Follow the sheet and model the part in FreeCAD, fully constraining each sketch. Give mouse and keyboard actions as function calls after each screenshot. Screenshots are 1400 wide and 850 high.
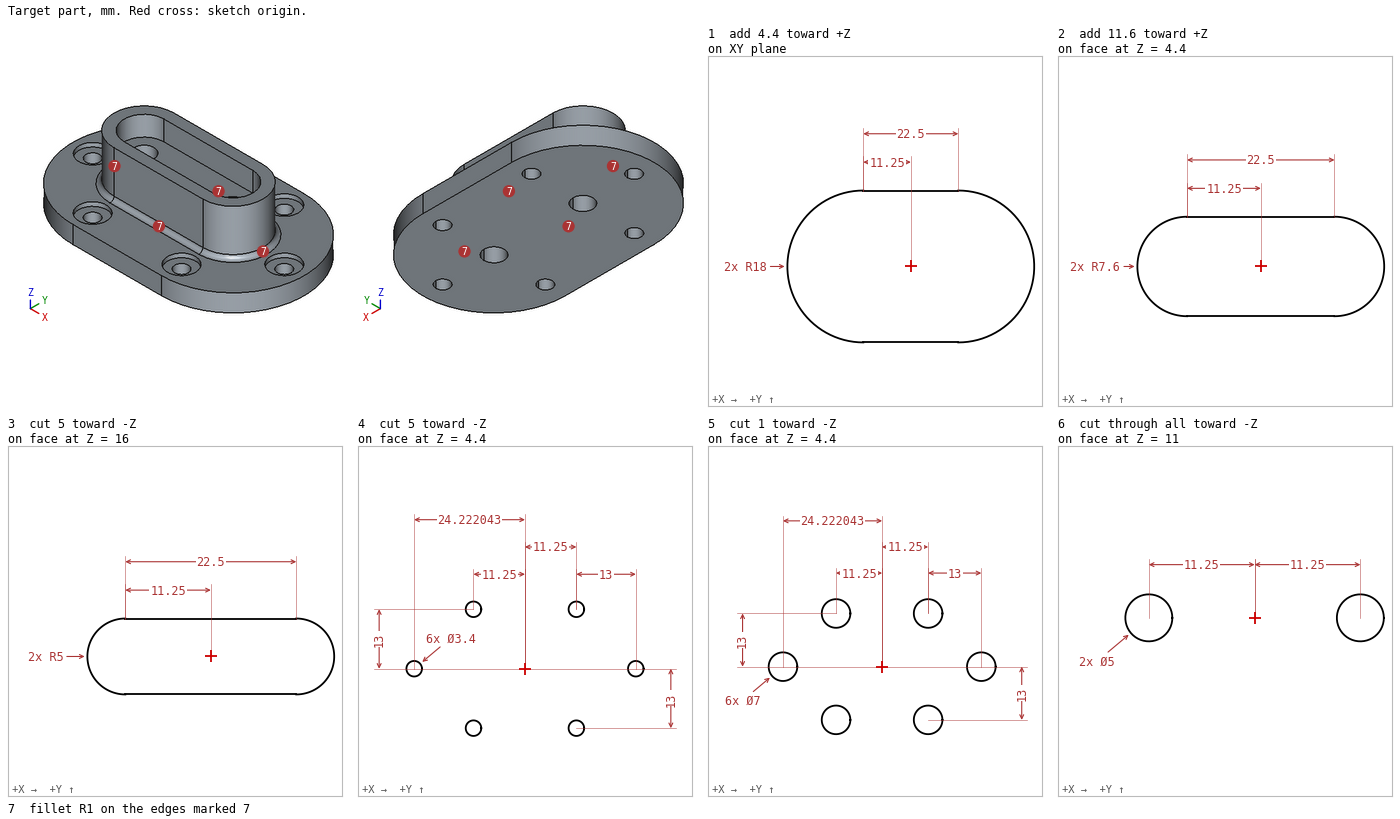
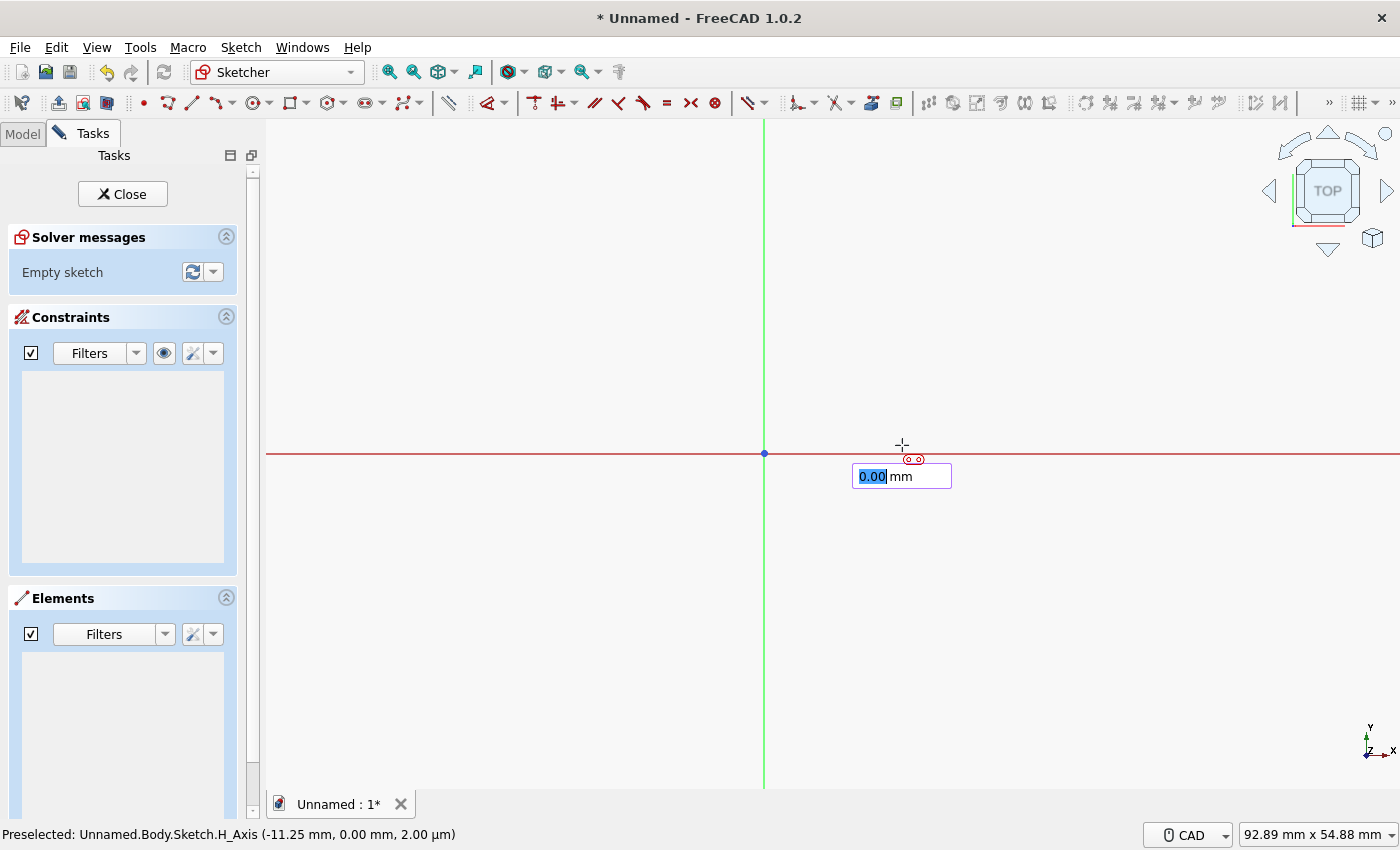
click(805, 234)
key(Escape)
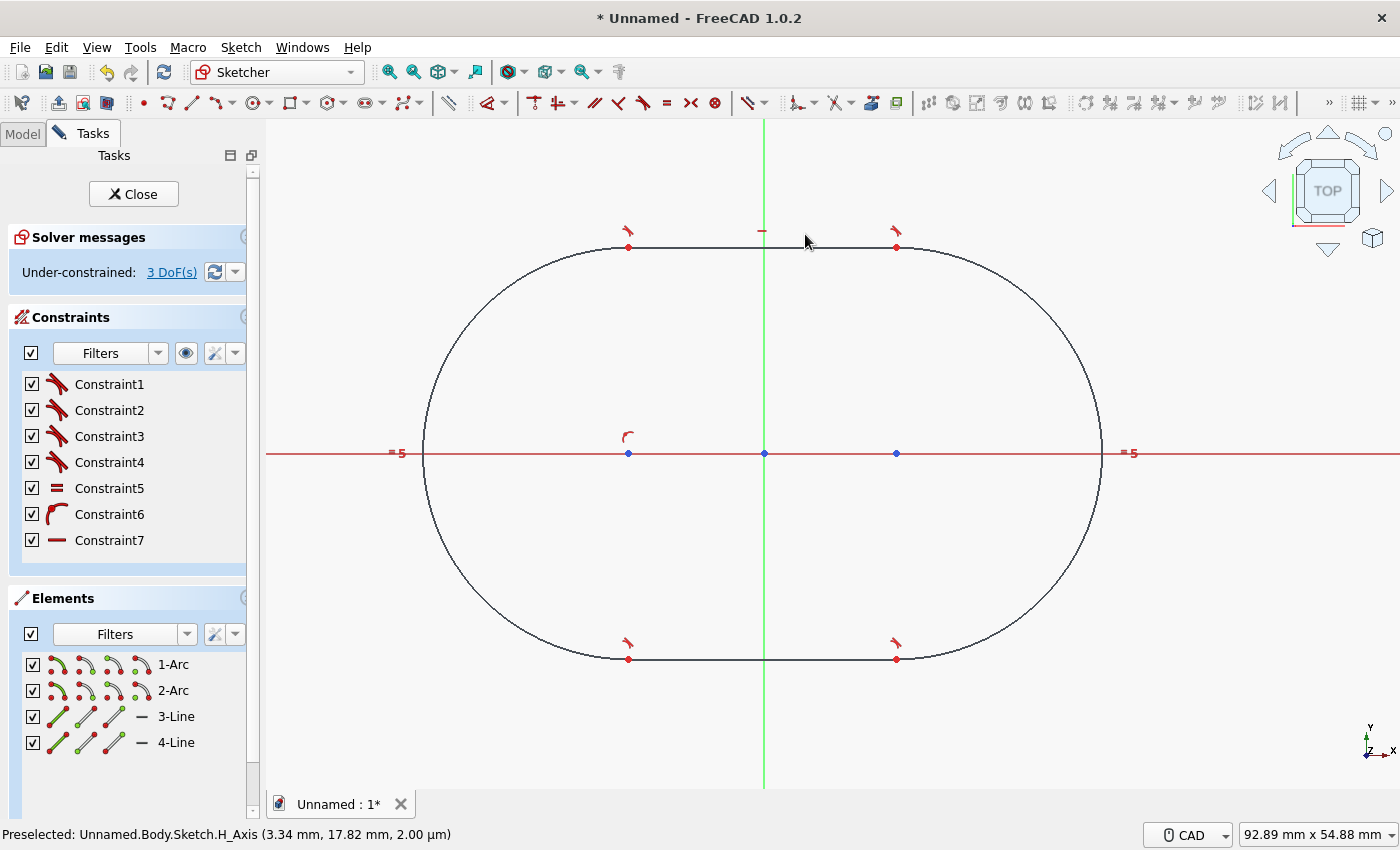
click(488, 104)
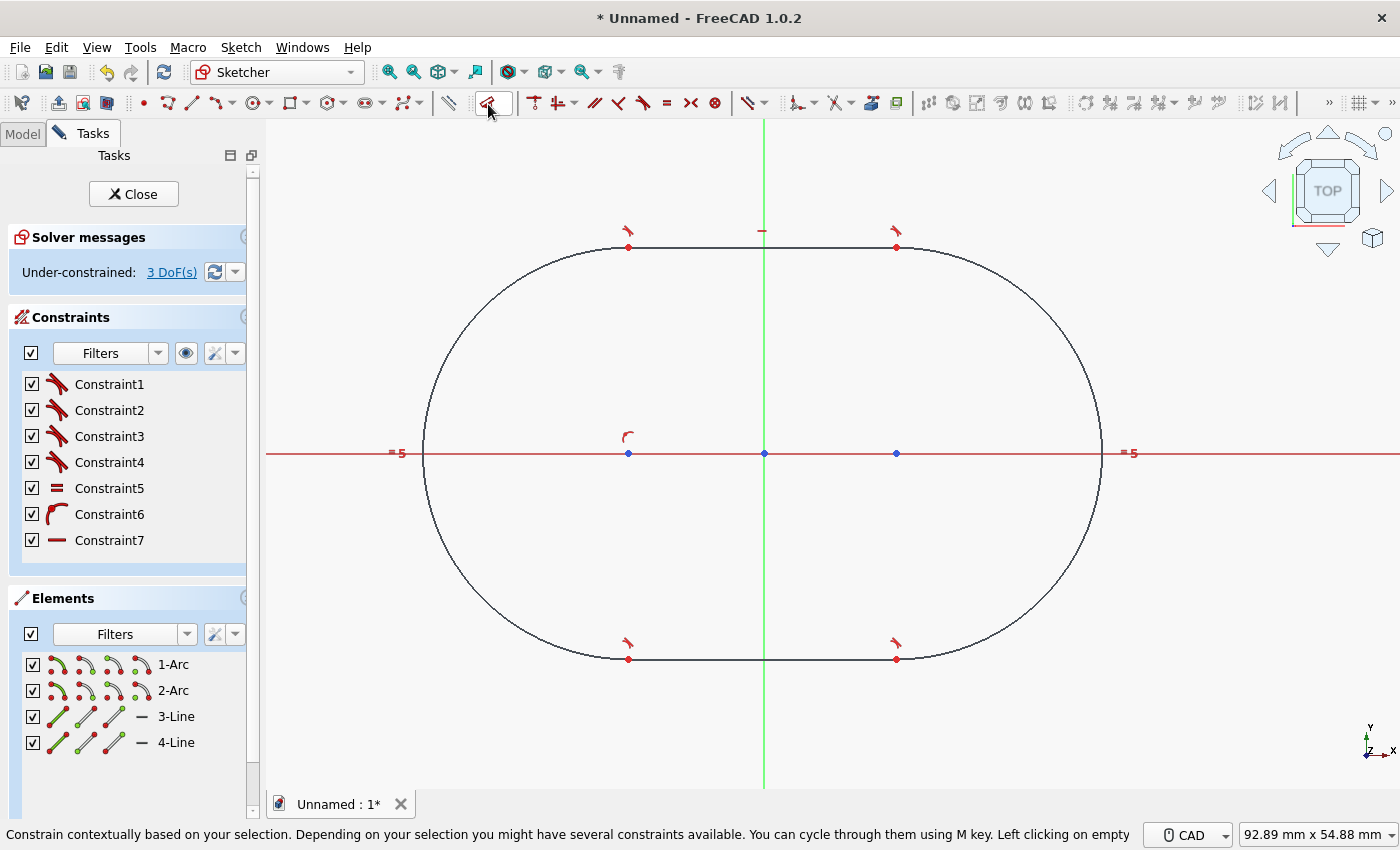
click(462, 333)
click(436, 314)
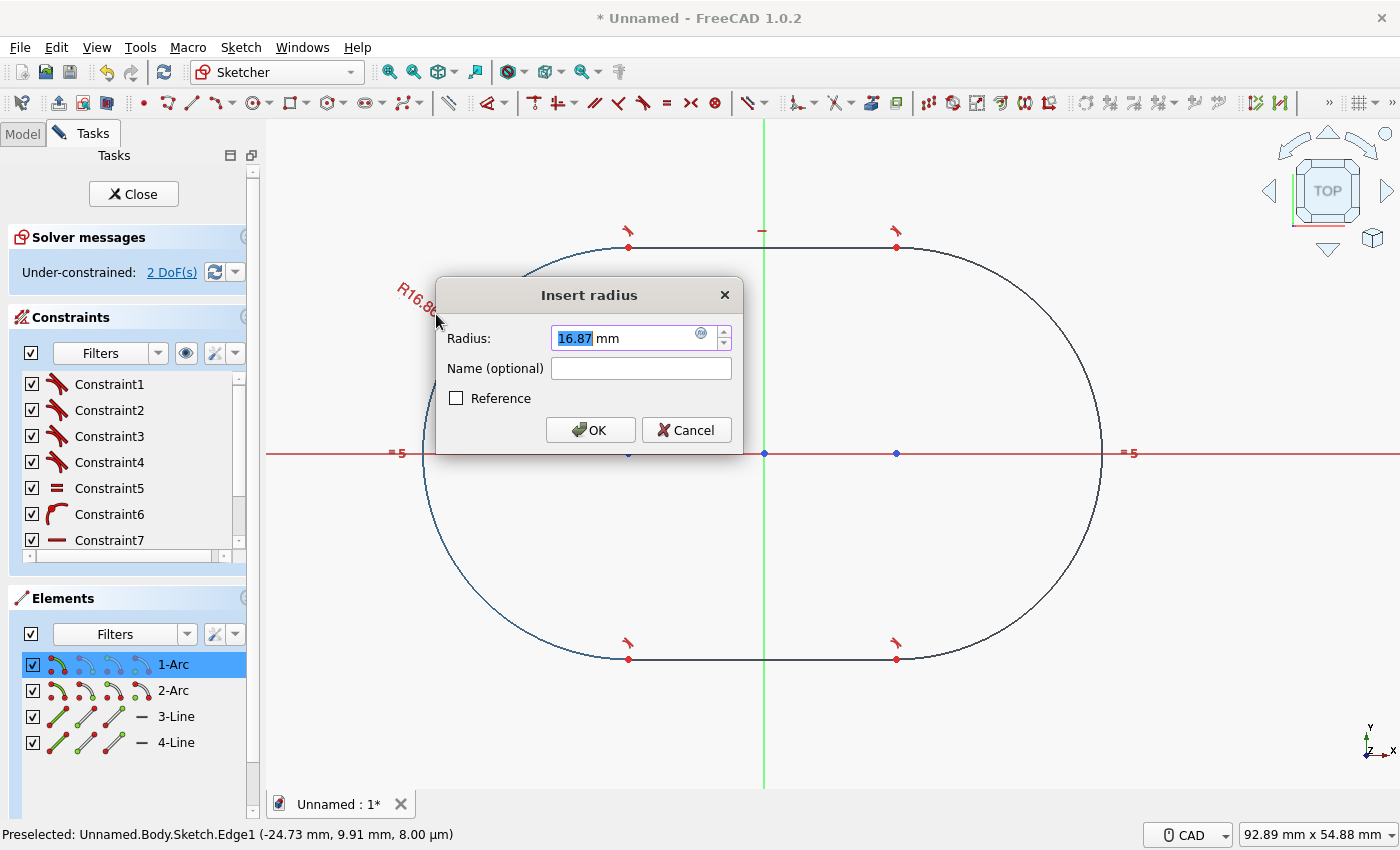
text(18)
key(Return)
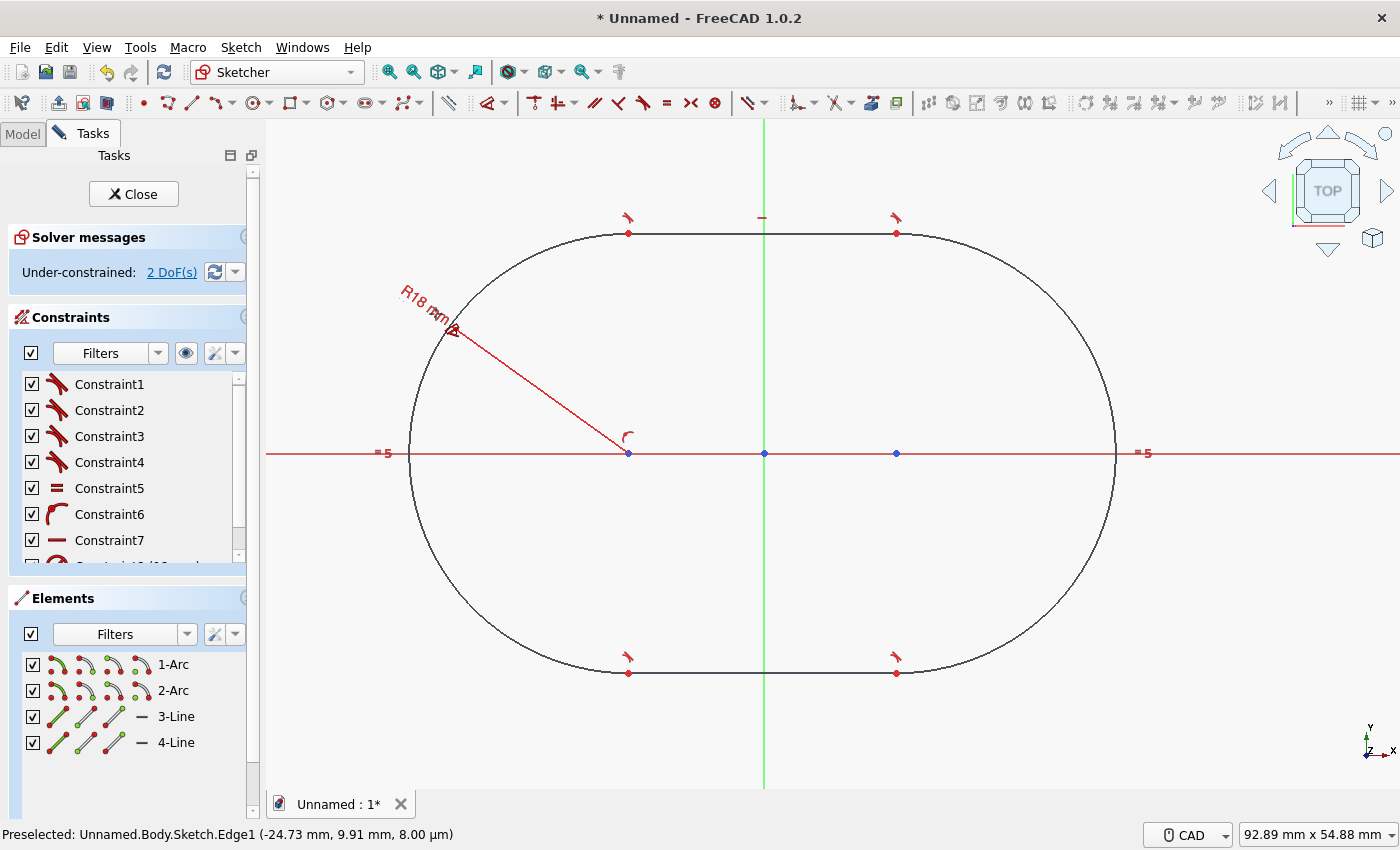
click(709, 234)
click(701, 200)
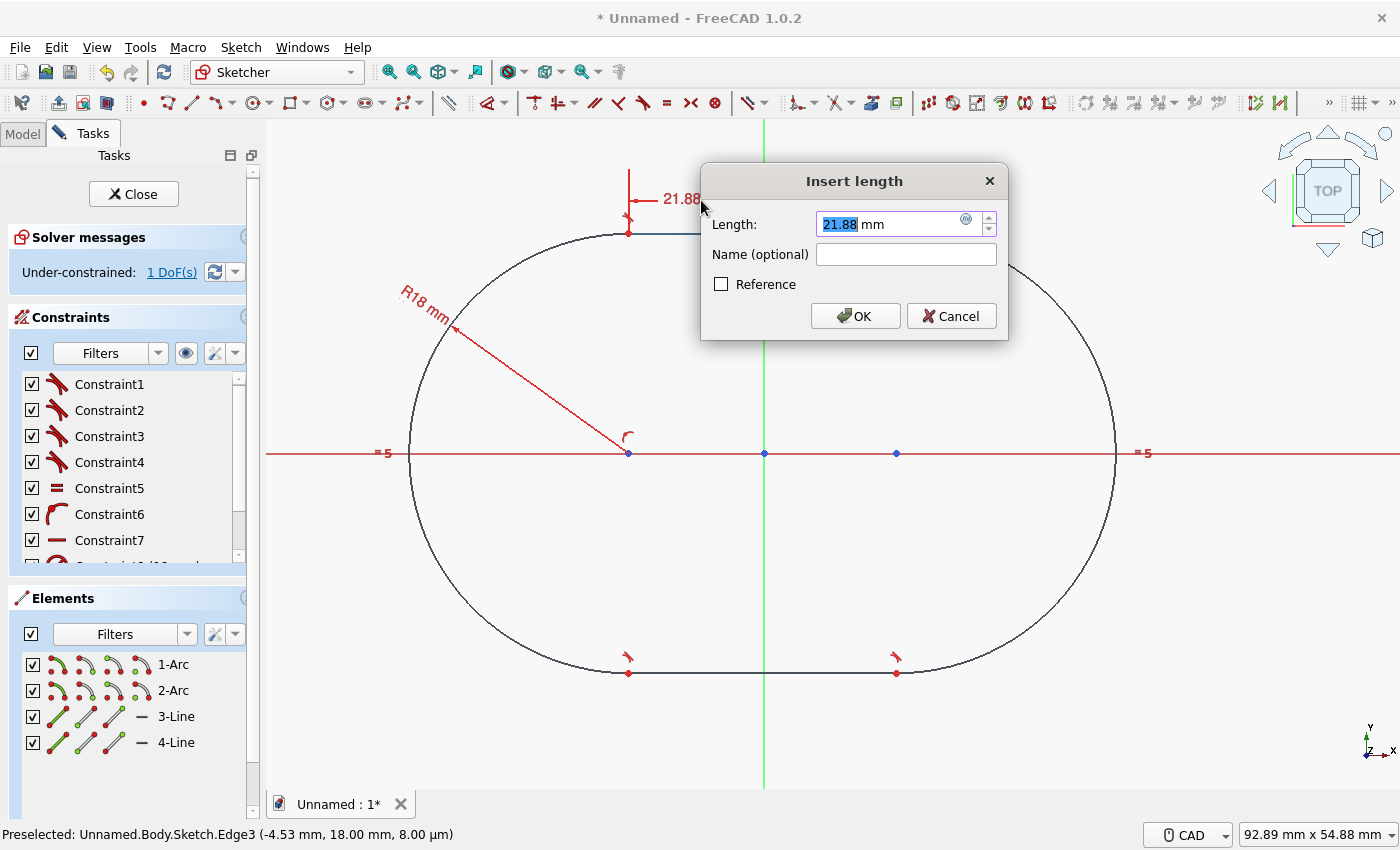
text(22.5)
key(Return)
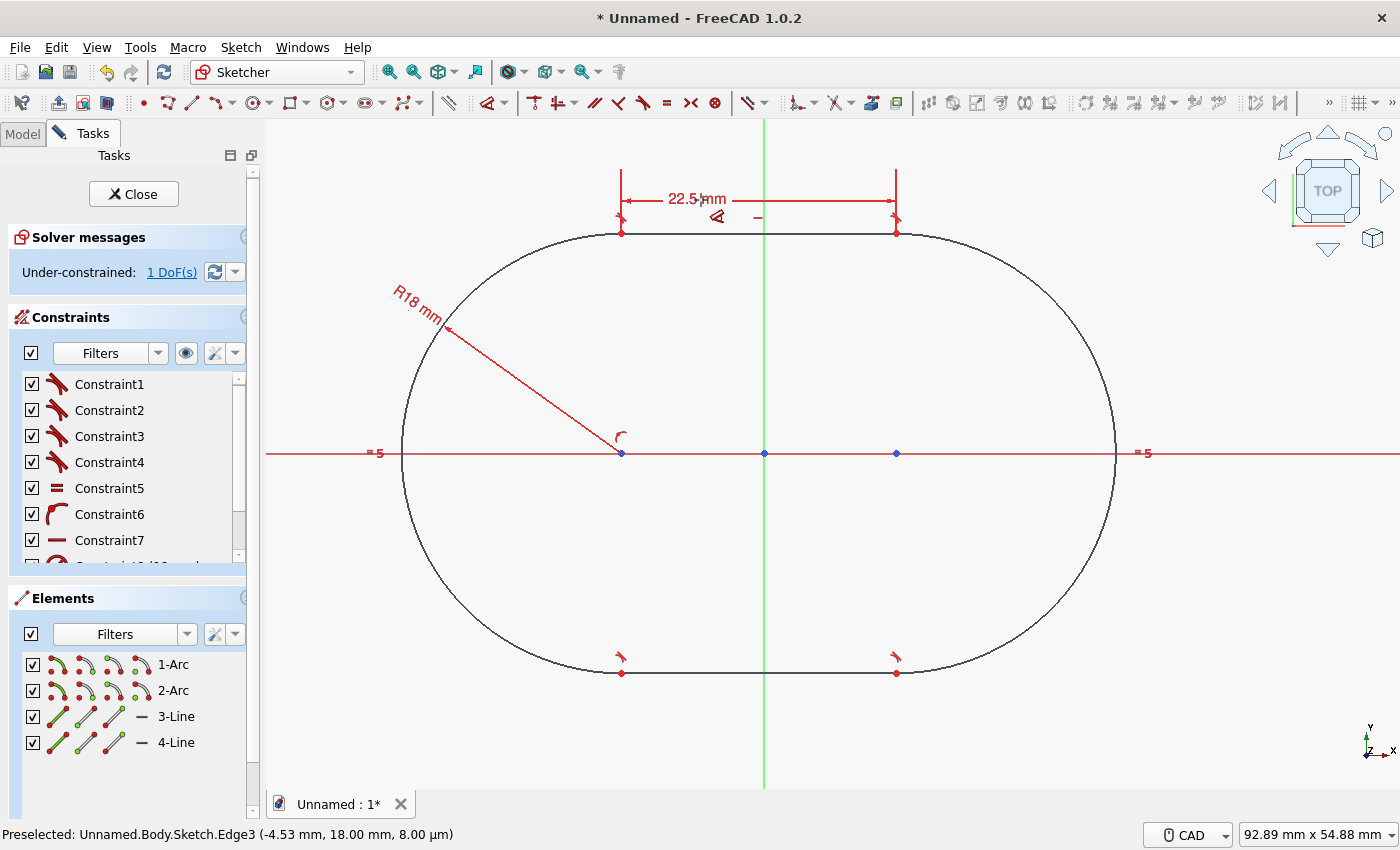
click(621, 234)
click(693, 488)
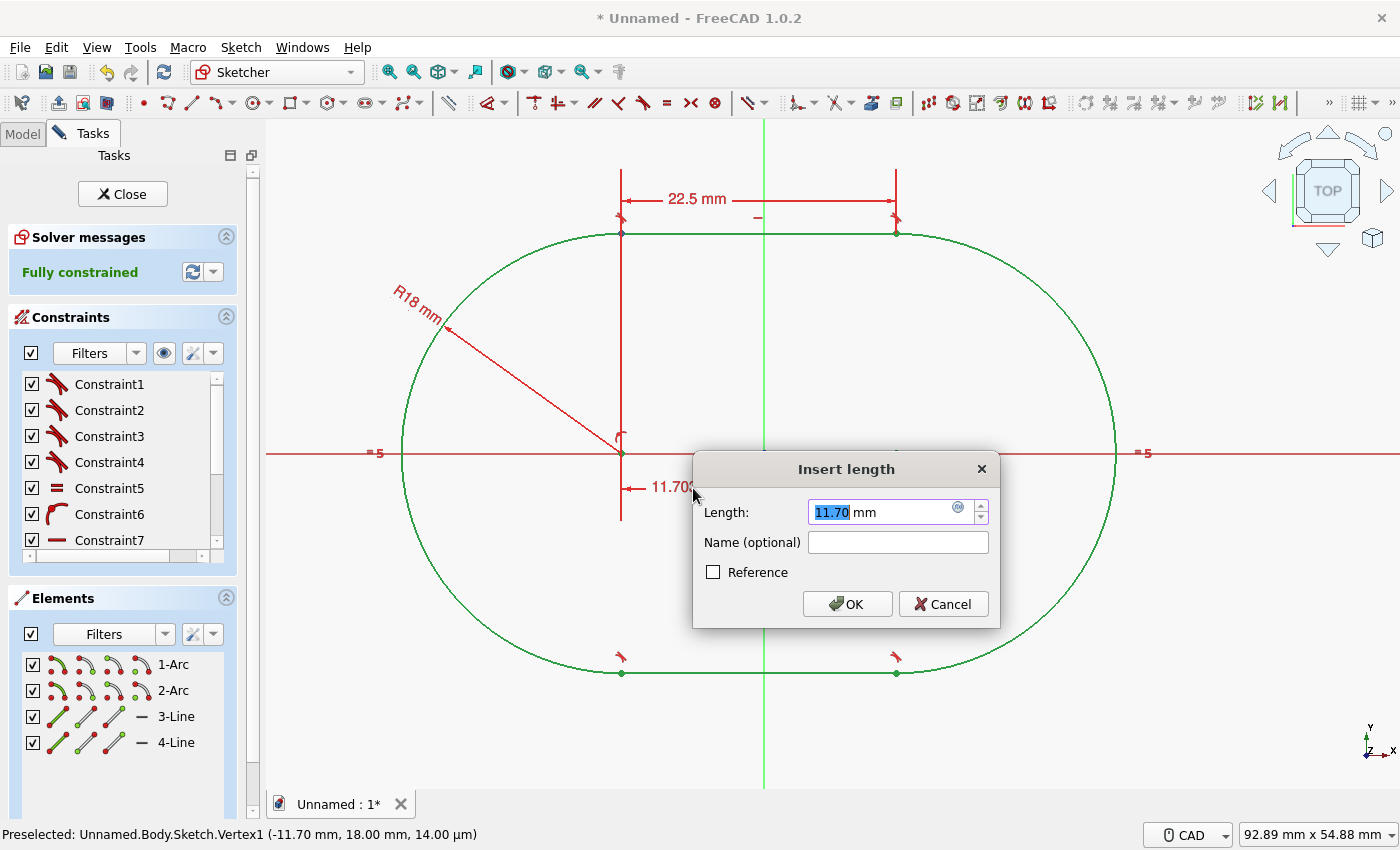
text(11.25)
key(Return)
key(Escape)